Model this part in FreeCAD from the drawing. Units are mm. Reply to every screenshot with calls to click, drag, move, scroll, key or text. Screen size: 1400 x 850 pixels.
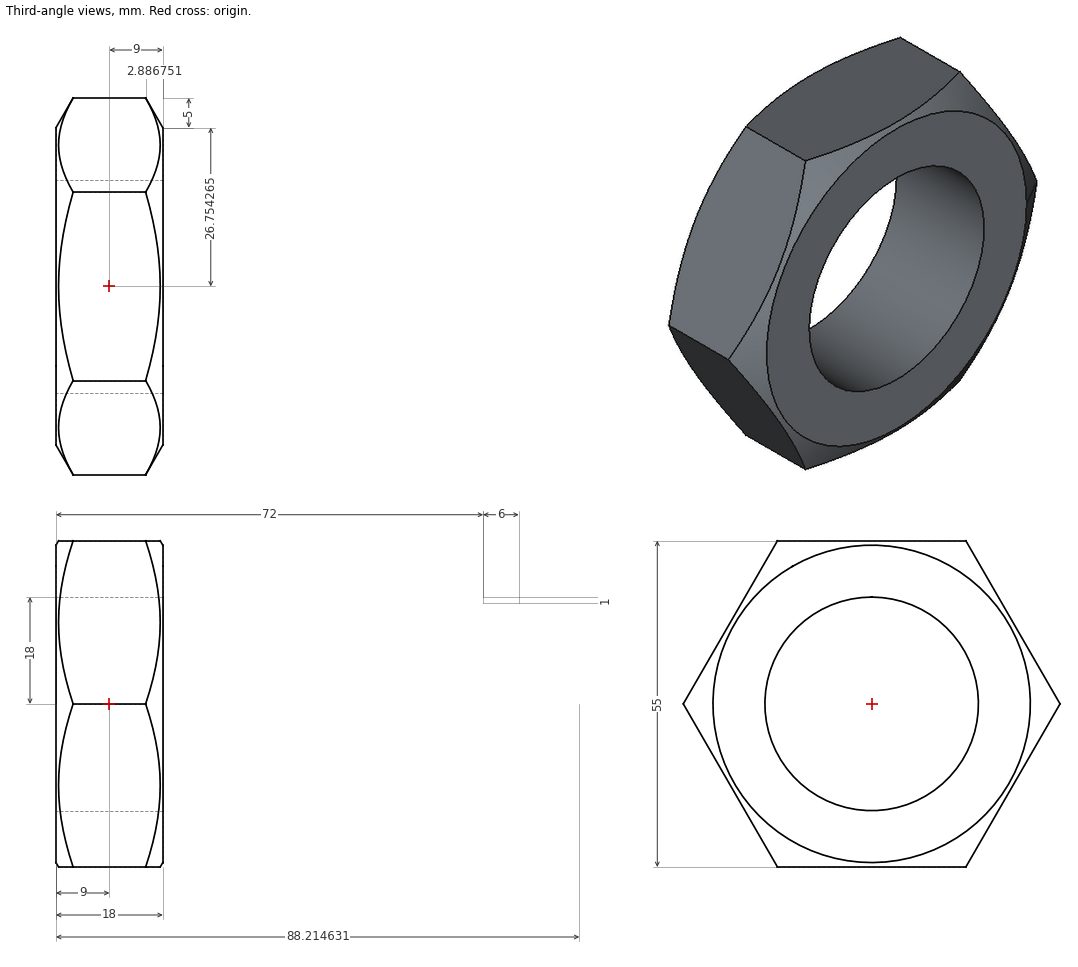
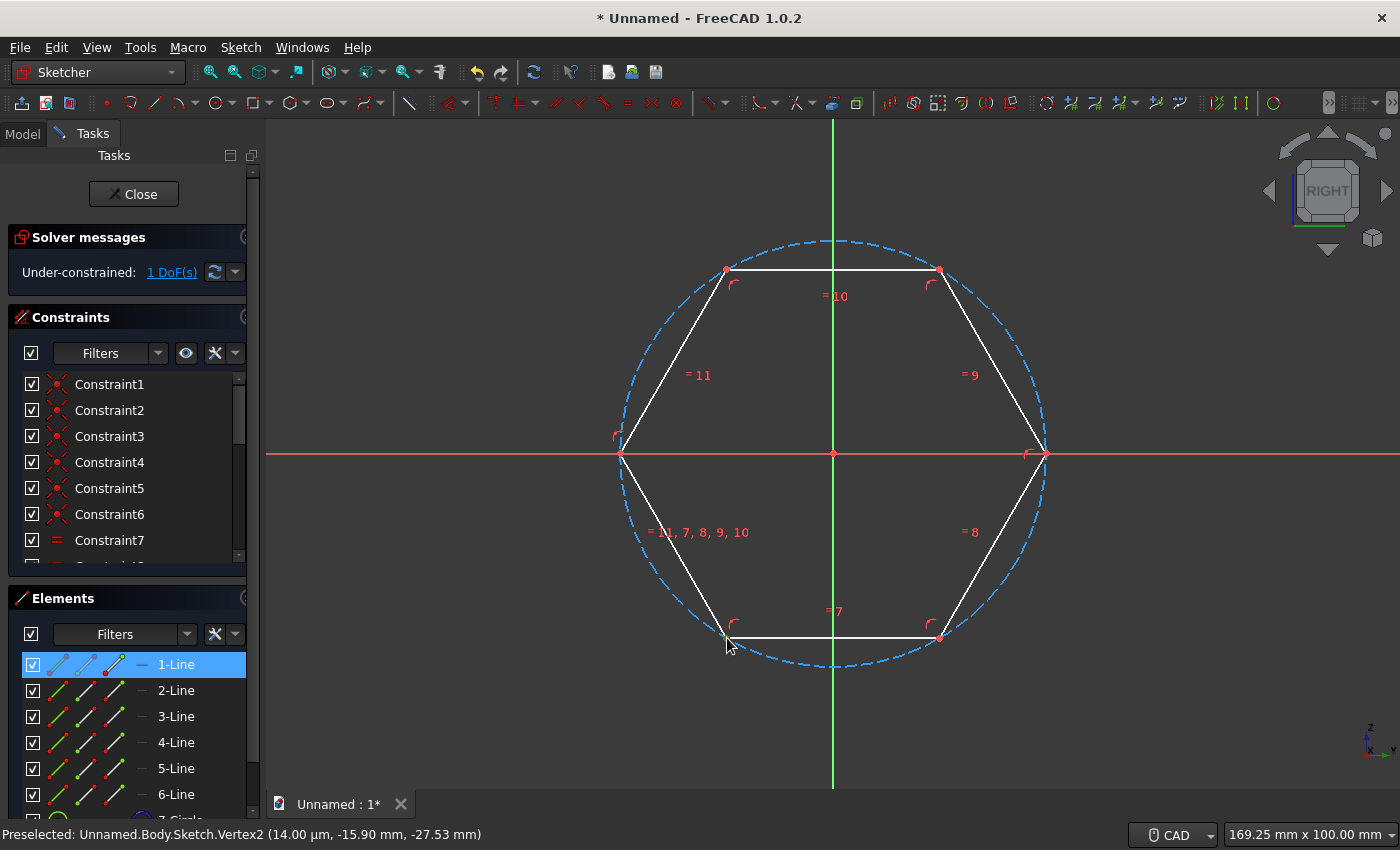
click(939, 270)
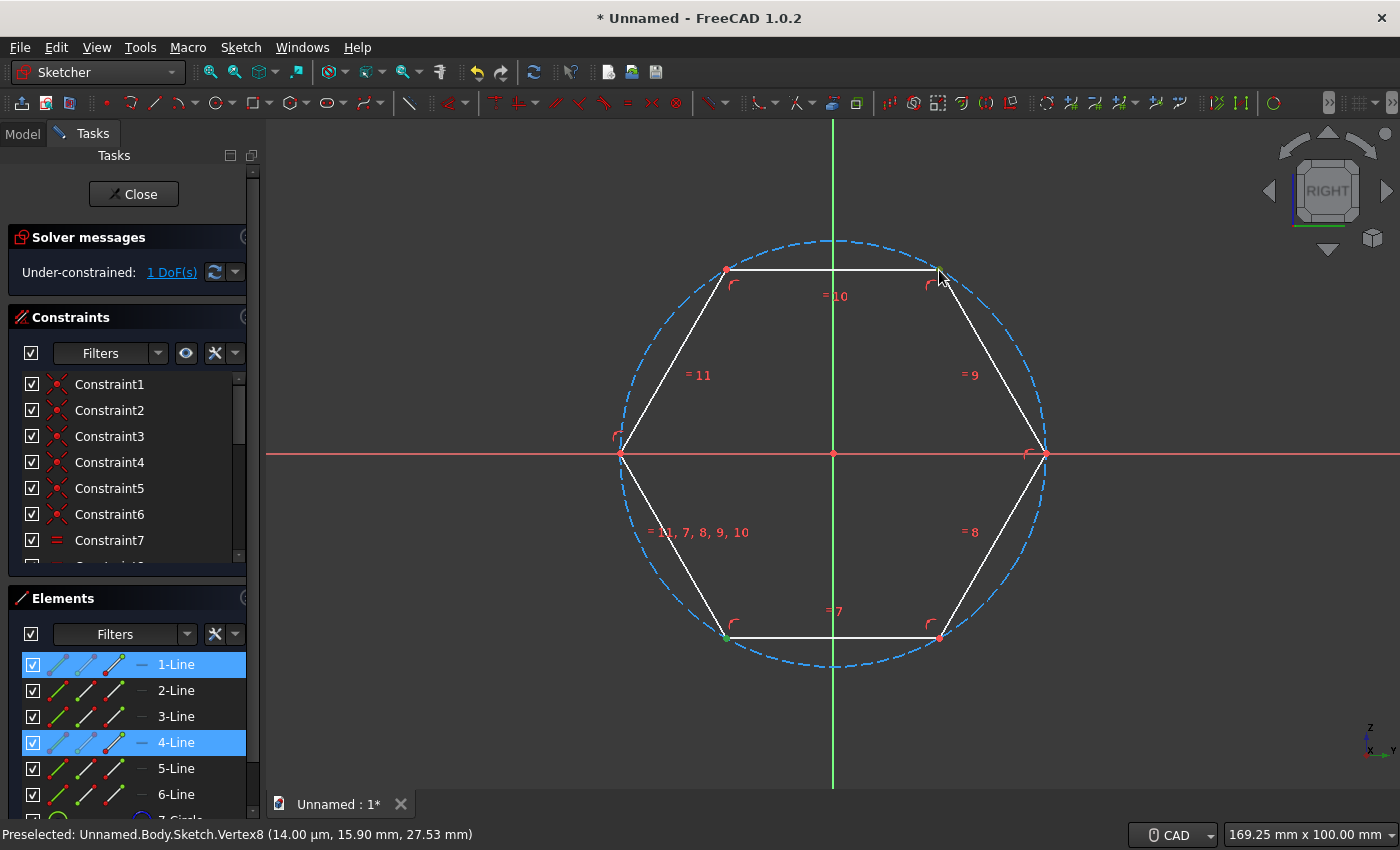
key(i)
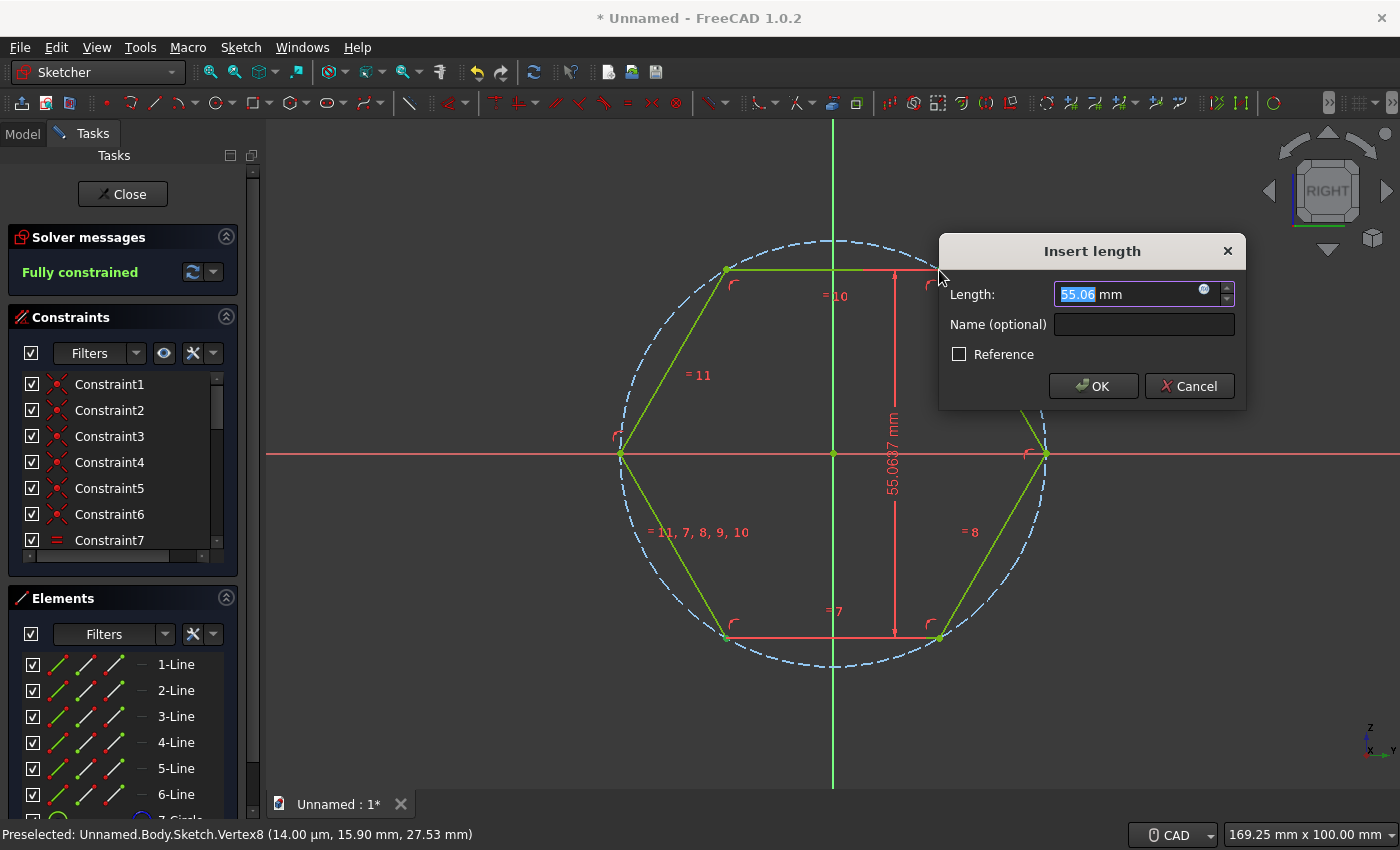
text(55)
key(Return)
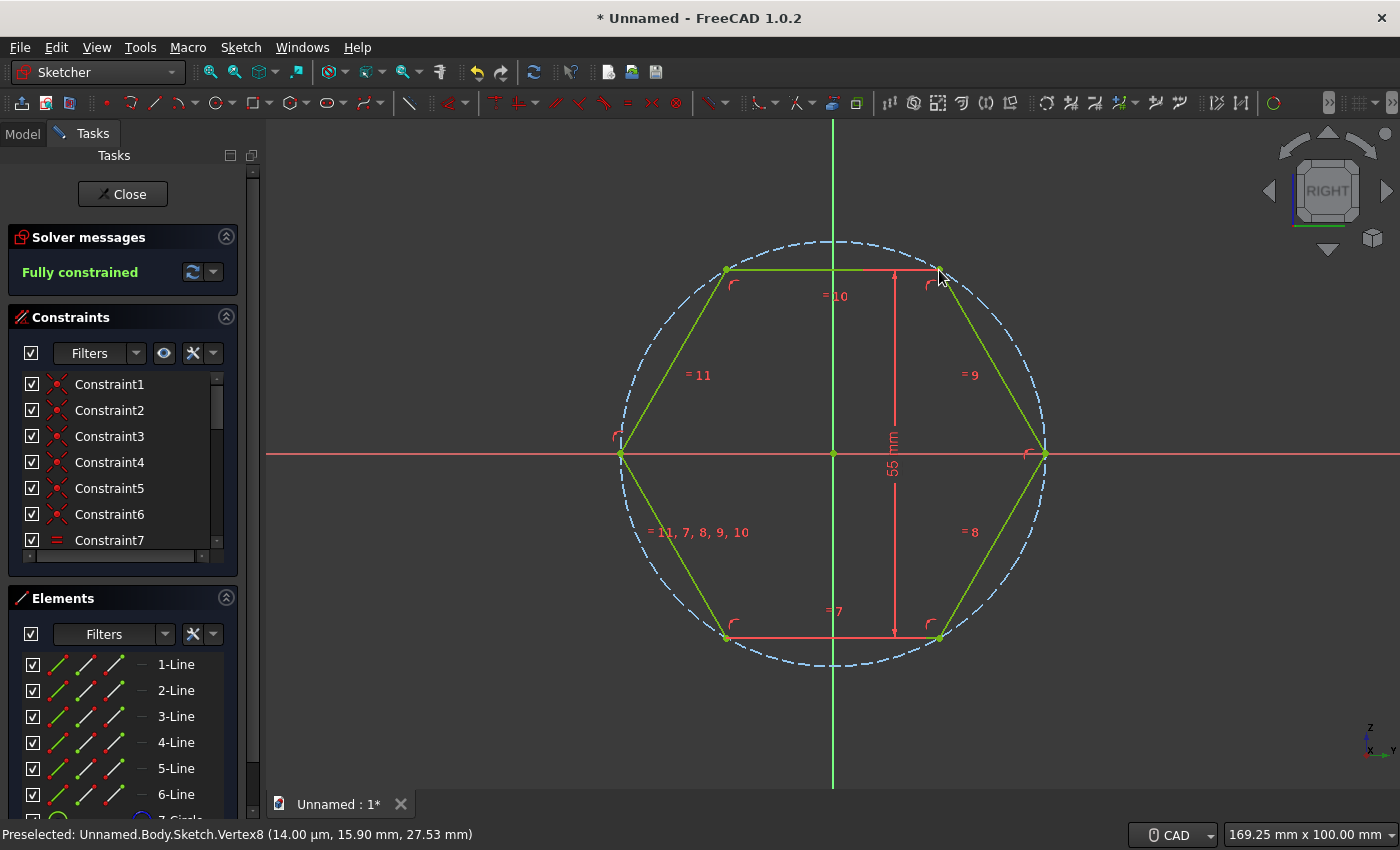
click(123, 194)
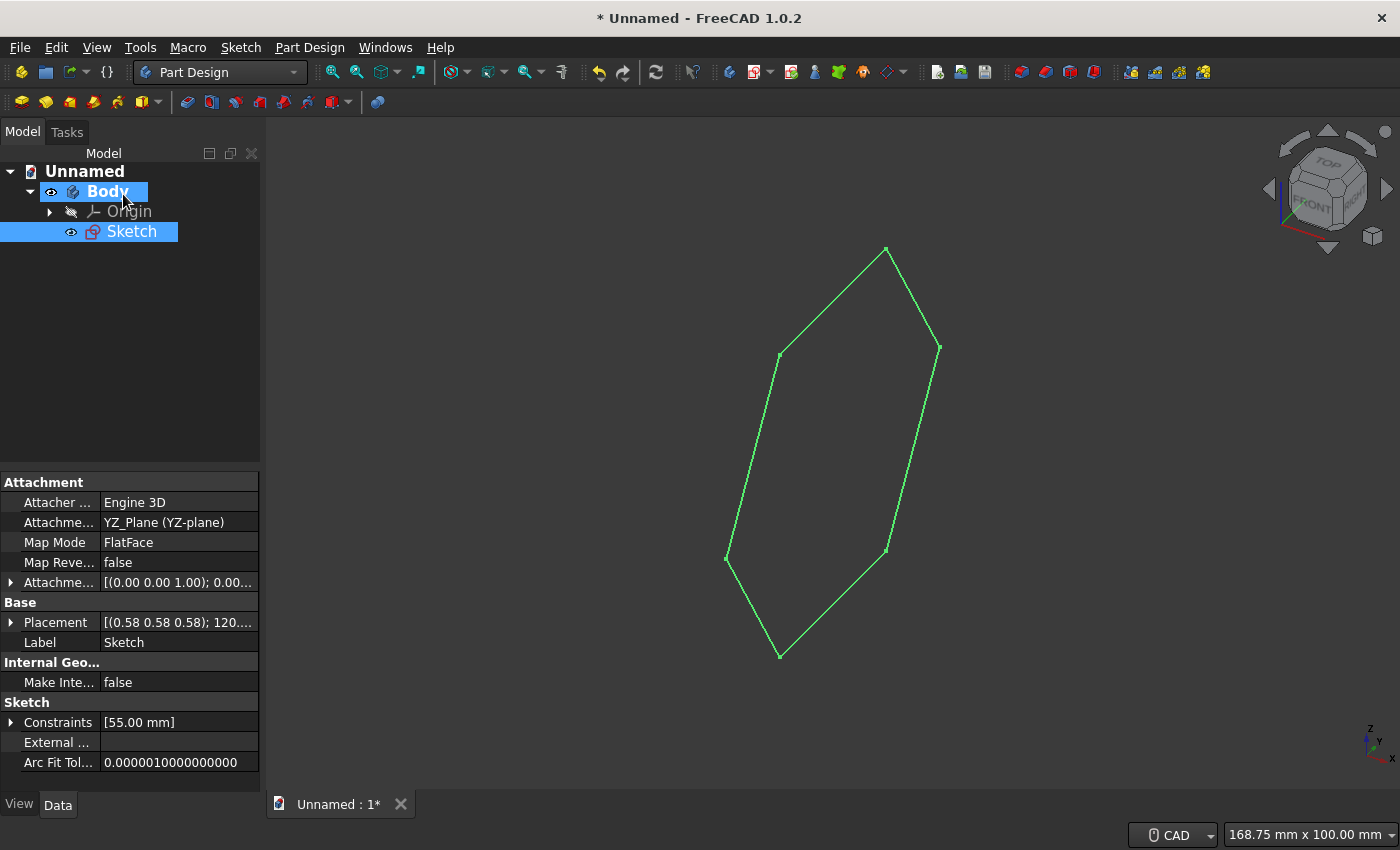
click(22, 102)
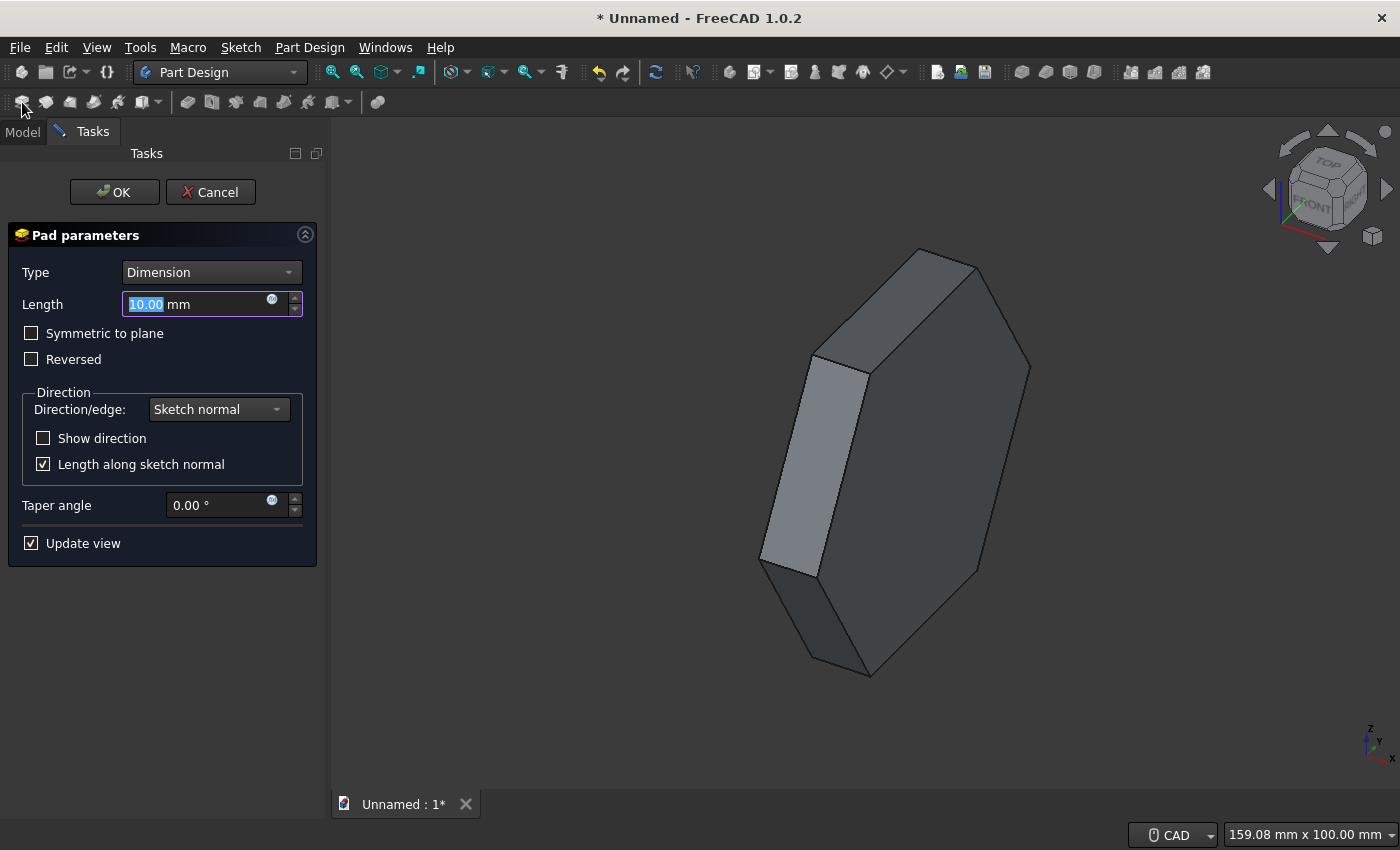
text(18)
key(Tab)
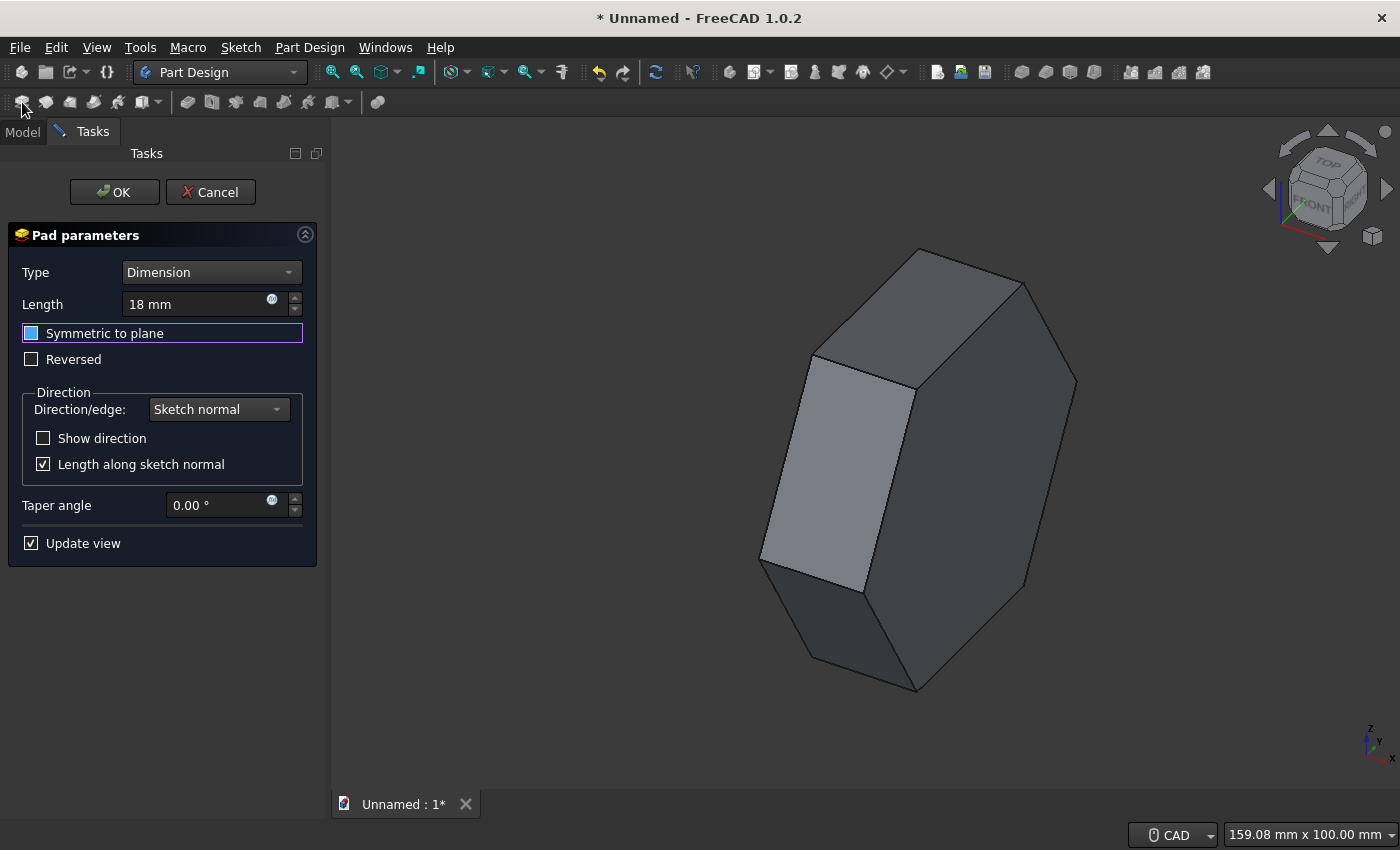
click(30, 333)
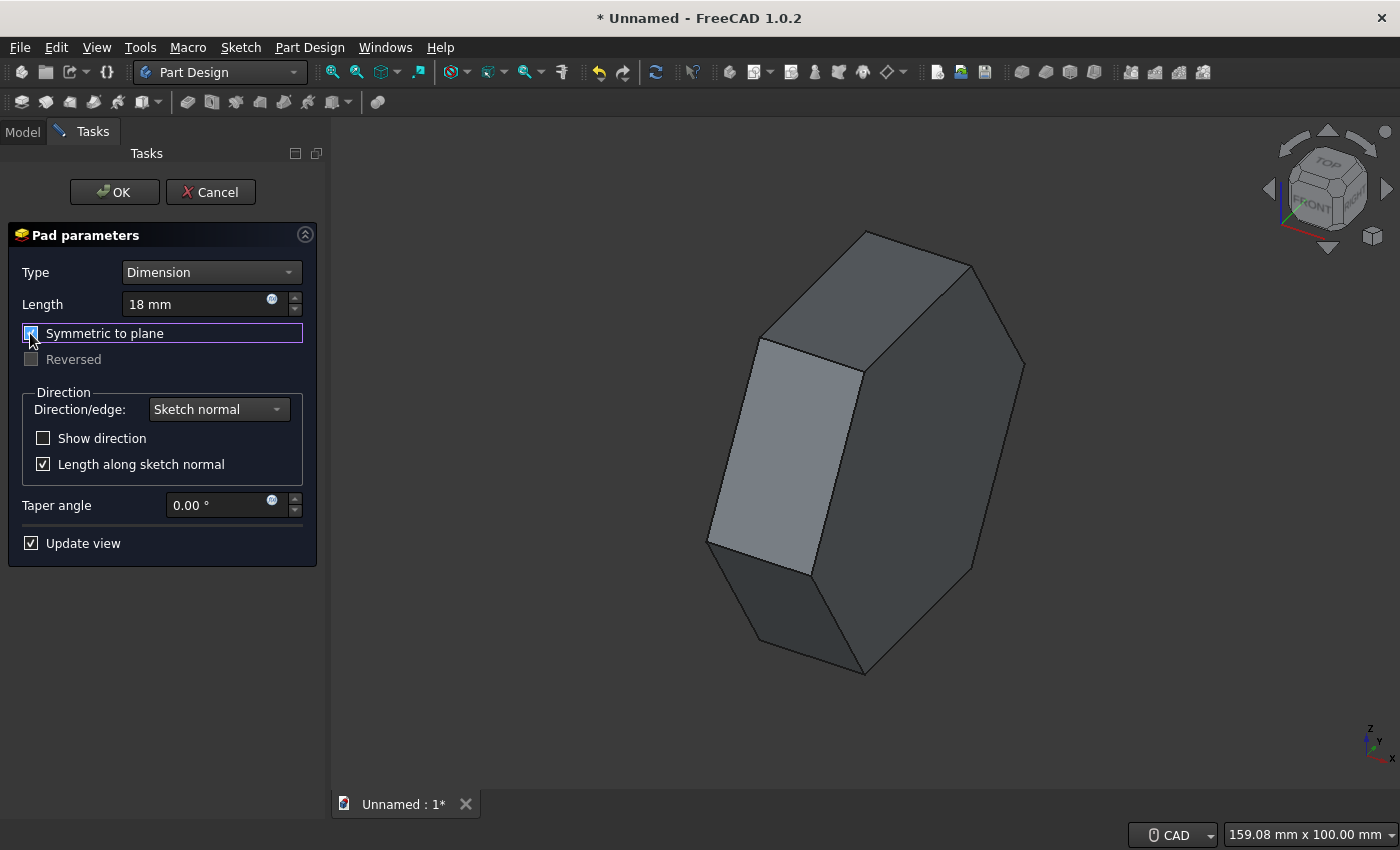
click(115, 192)